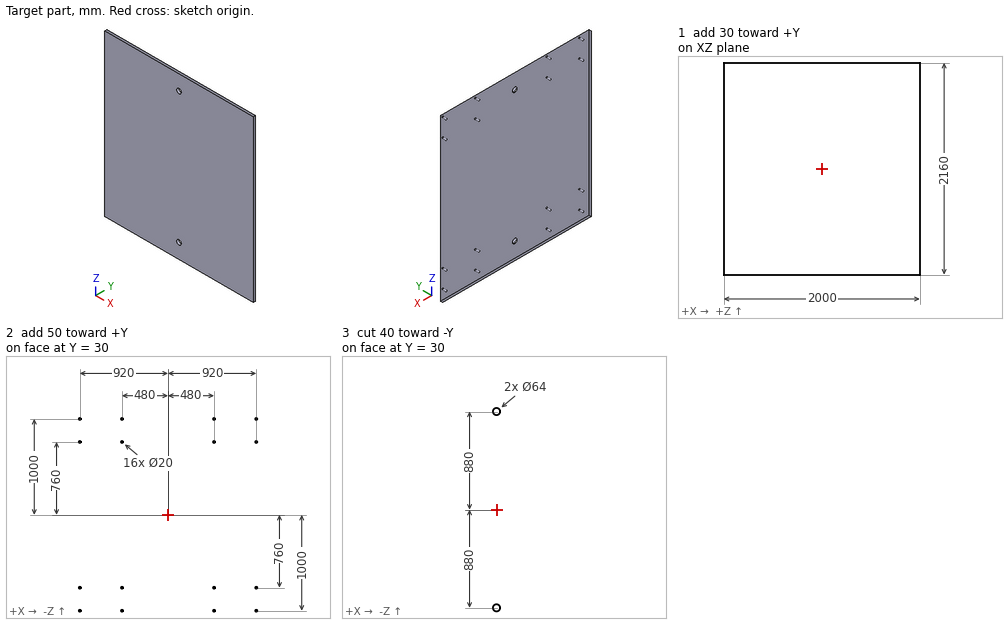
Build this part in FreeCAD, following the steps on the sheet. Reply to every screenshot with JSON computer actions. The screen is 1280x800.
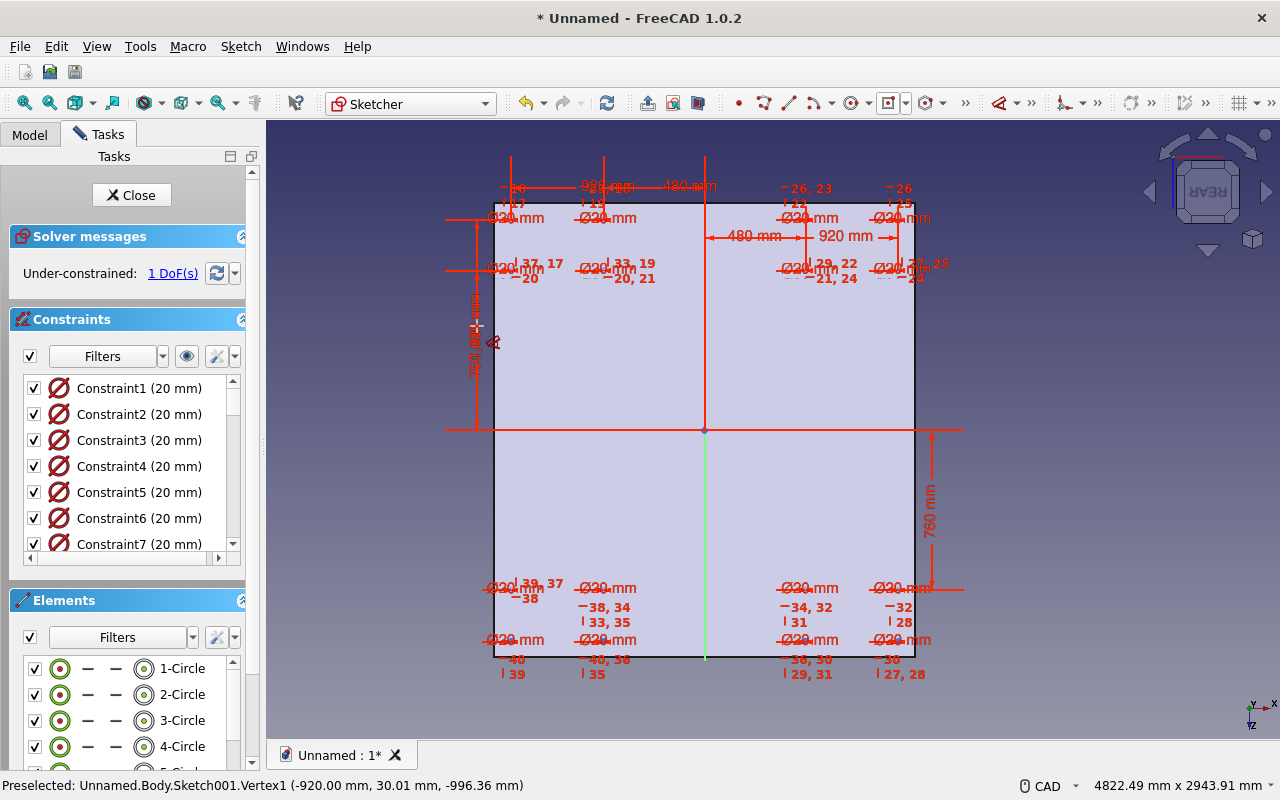
{"action": "left_click", "coordinate": [898, 642]}
{"action": "left_click", "coordinate": [932, 536]}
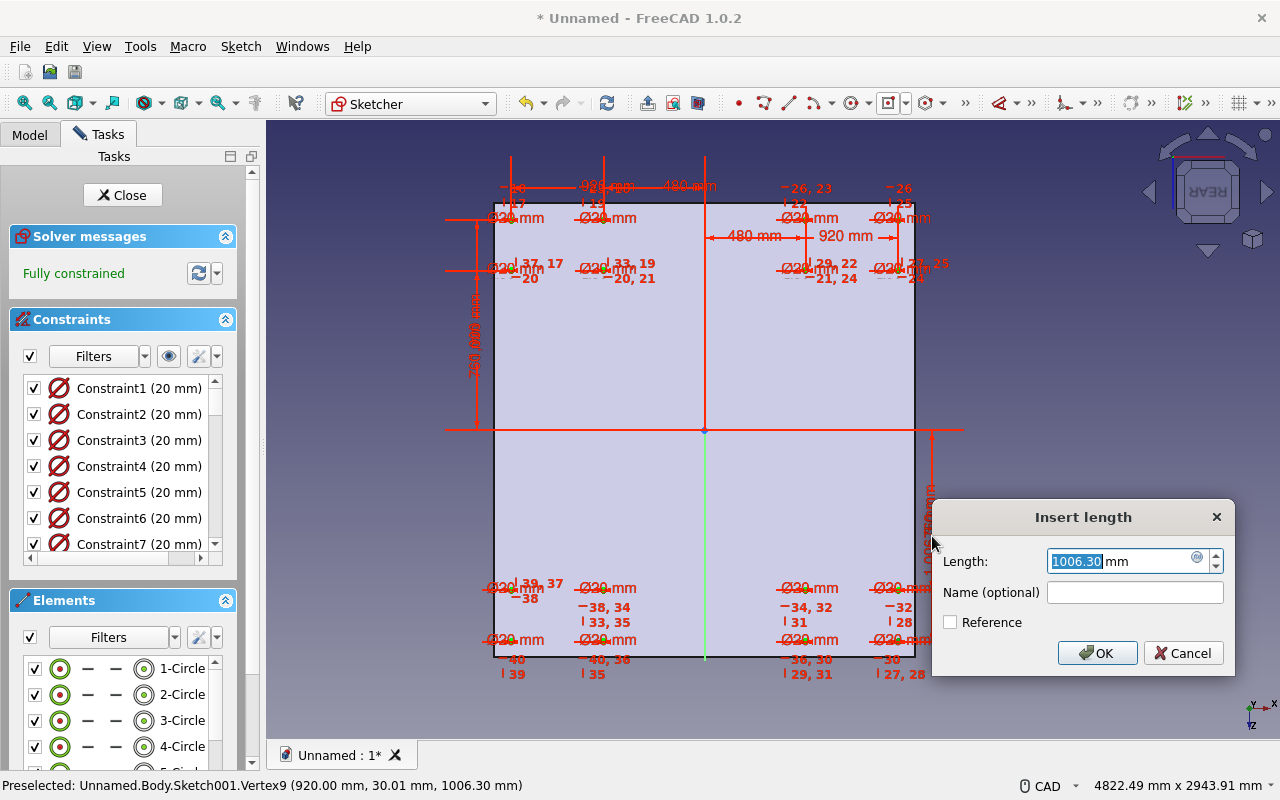
{"action": "type", "text": "1000"}
{"action": "key", "text": "Return"}
{"action": "key", "text": "Escape"}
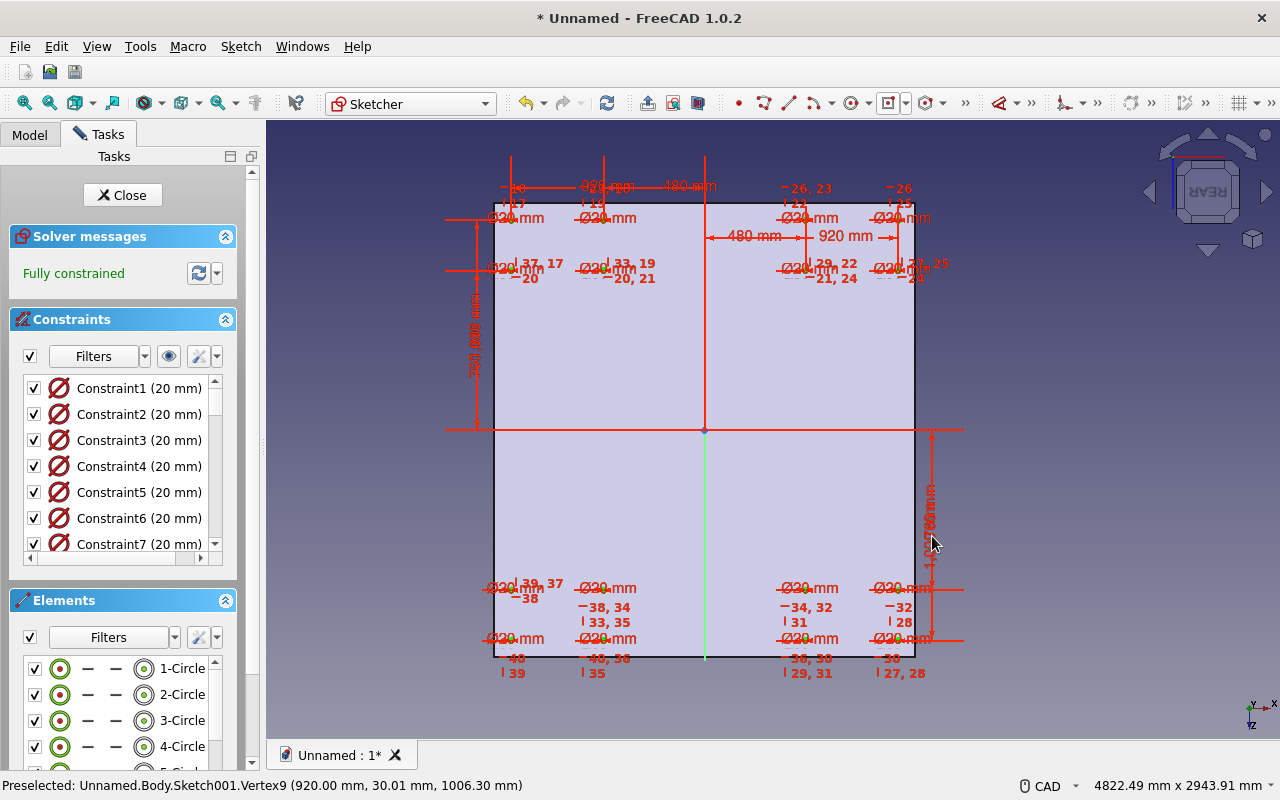
{"action": "left_click", "coordinate": [123, 195]}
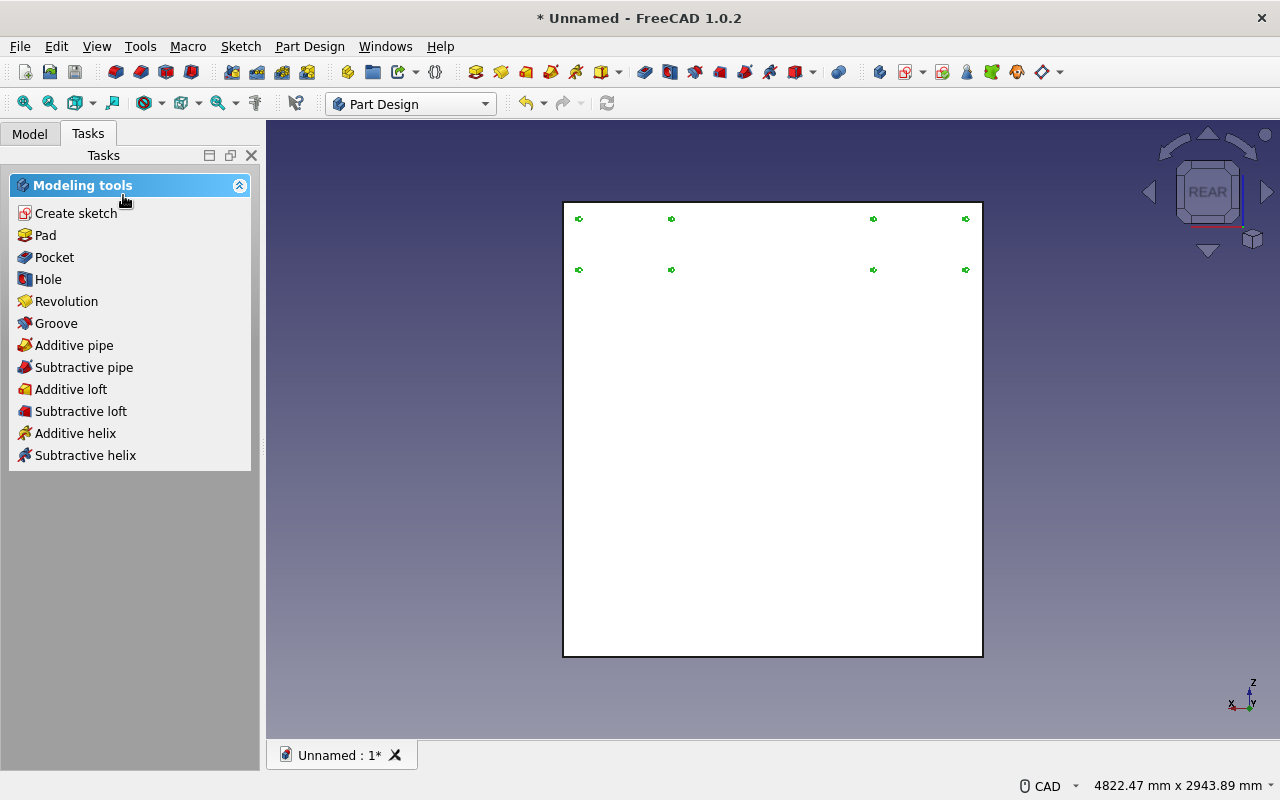
{"action": "left_click", "coordinate": [476, 72]}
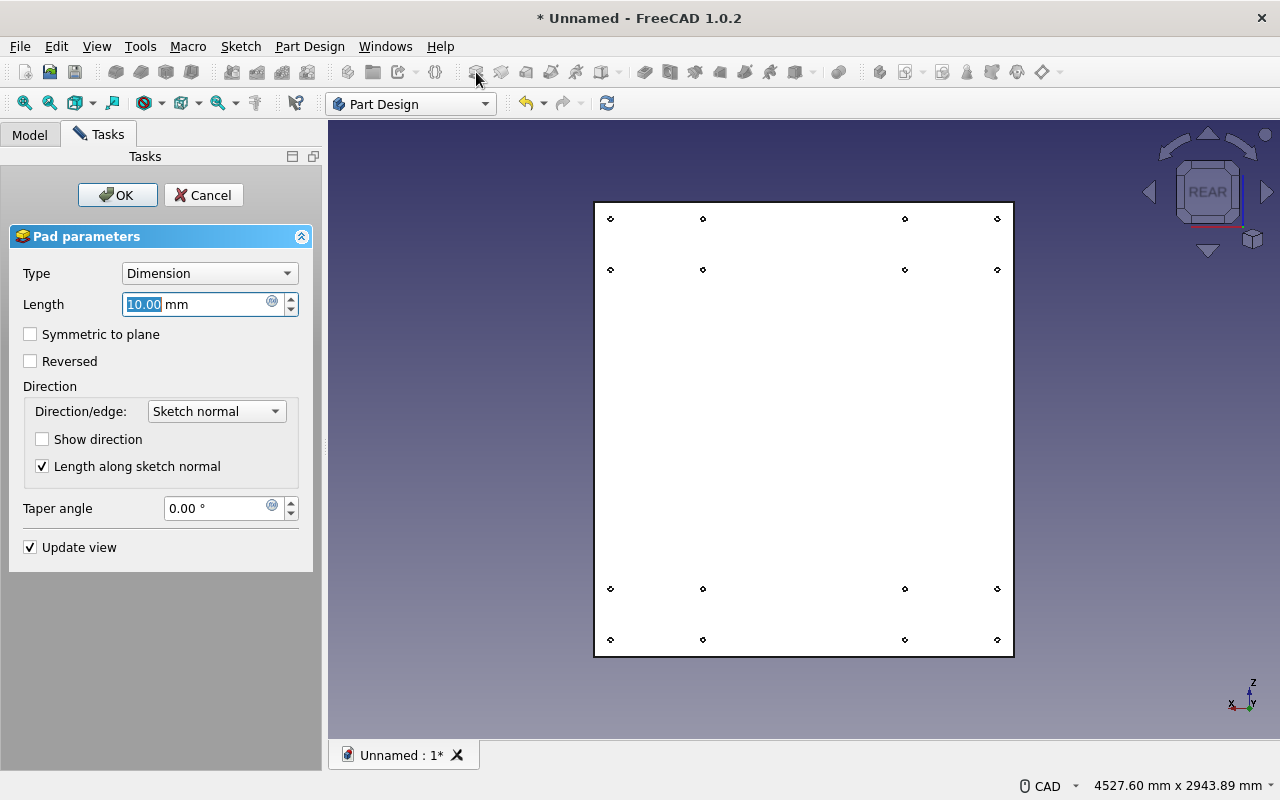
{"action": "type", "text": "50"}
{"action": "key", "text": "Tab"}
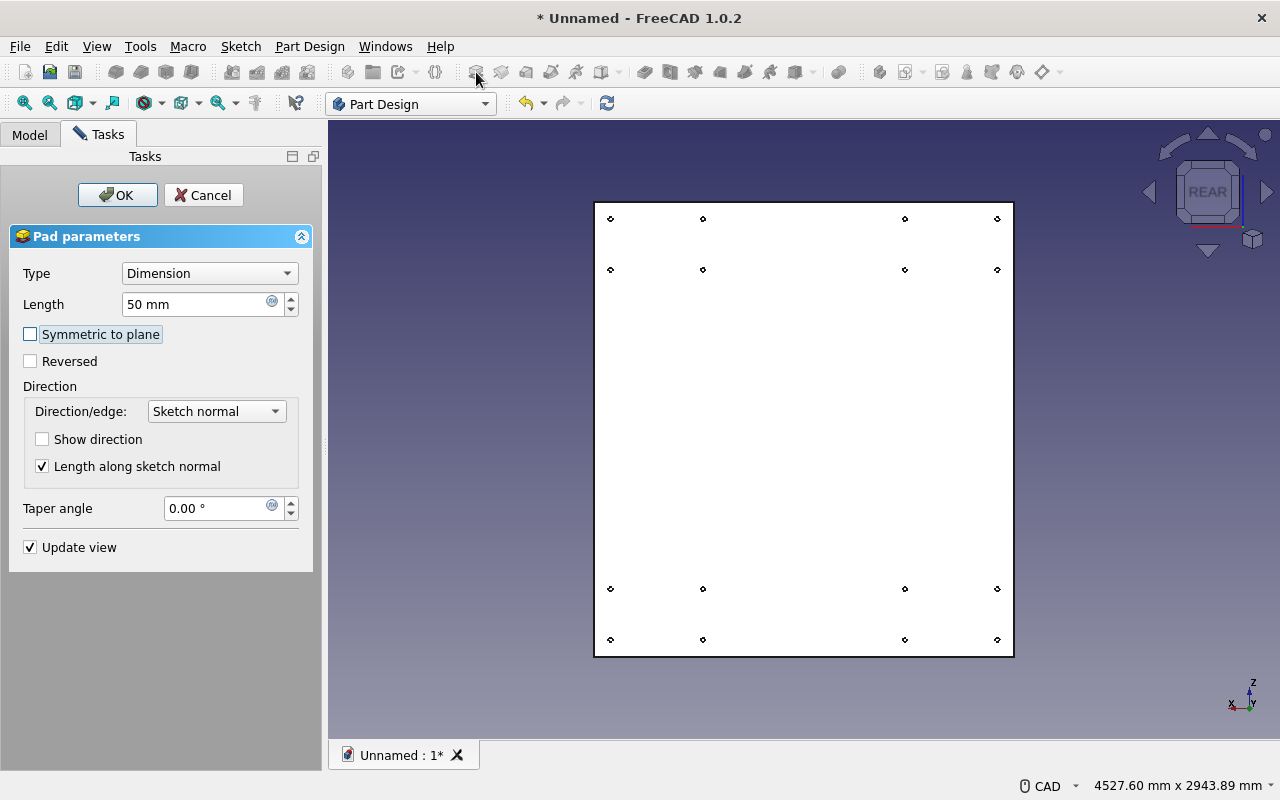
{"action": "left_click", "coordinate": [118, 195]}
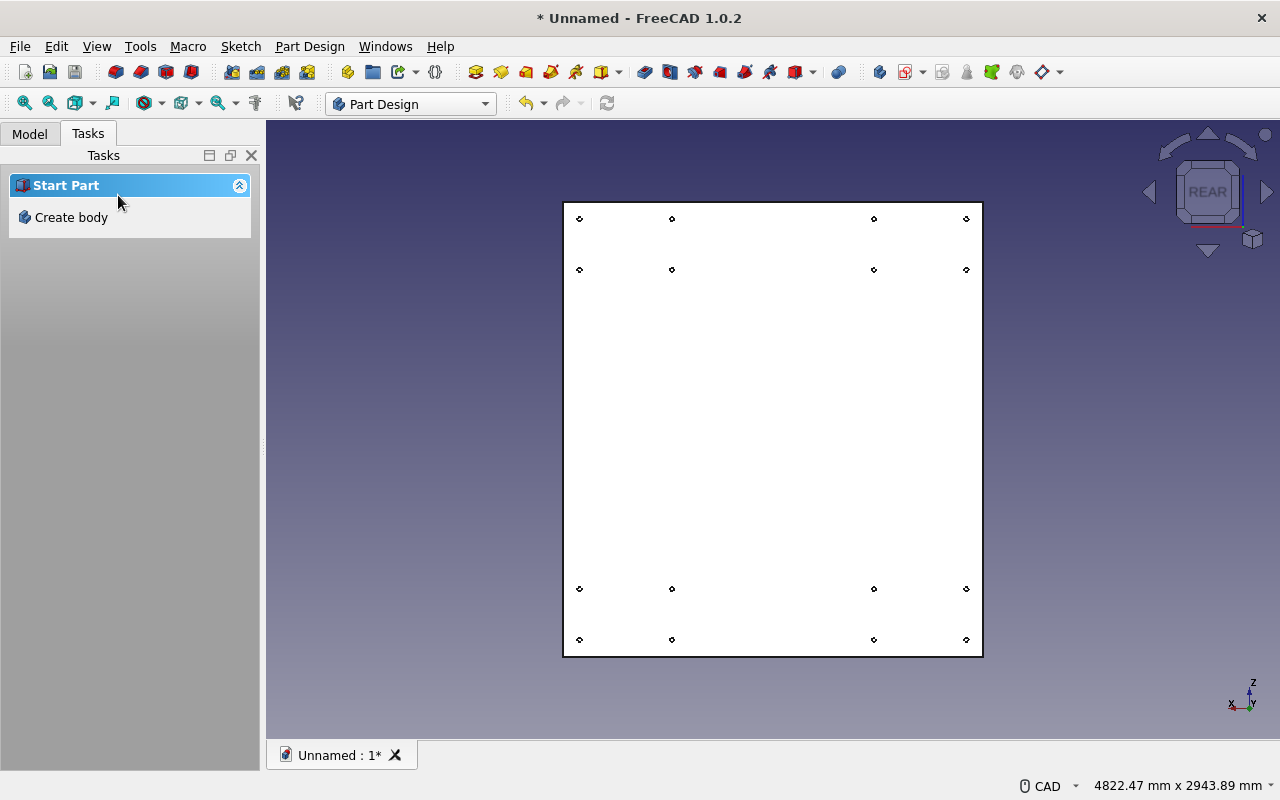
{"action": "left_click", "coordinate": [773, 429]}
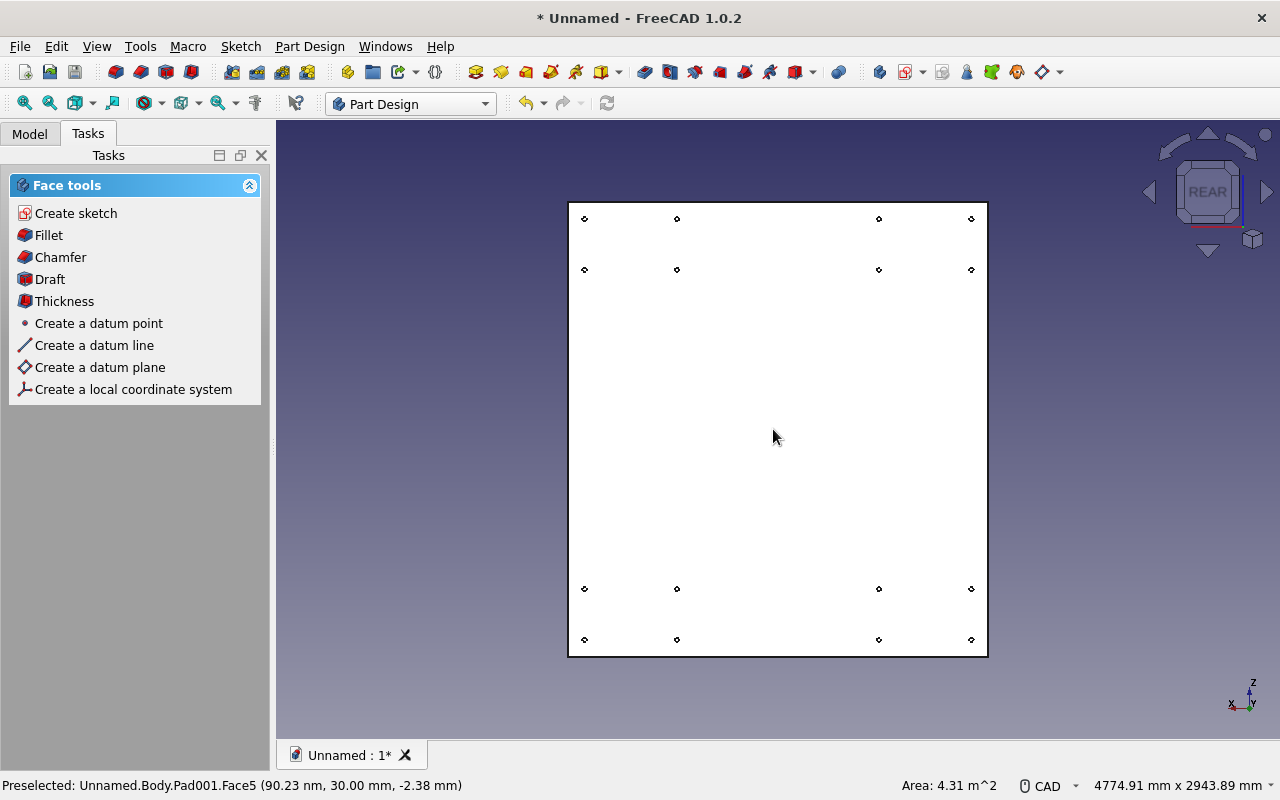
{"action": "left_click", "coordinate": [904, 72]}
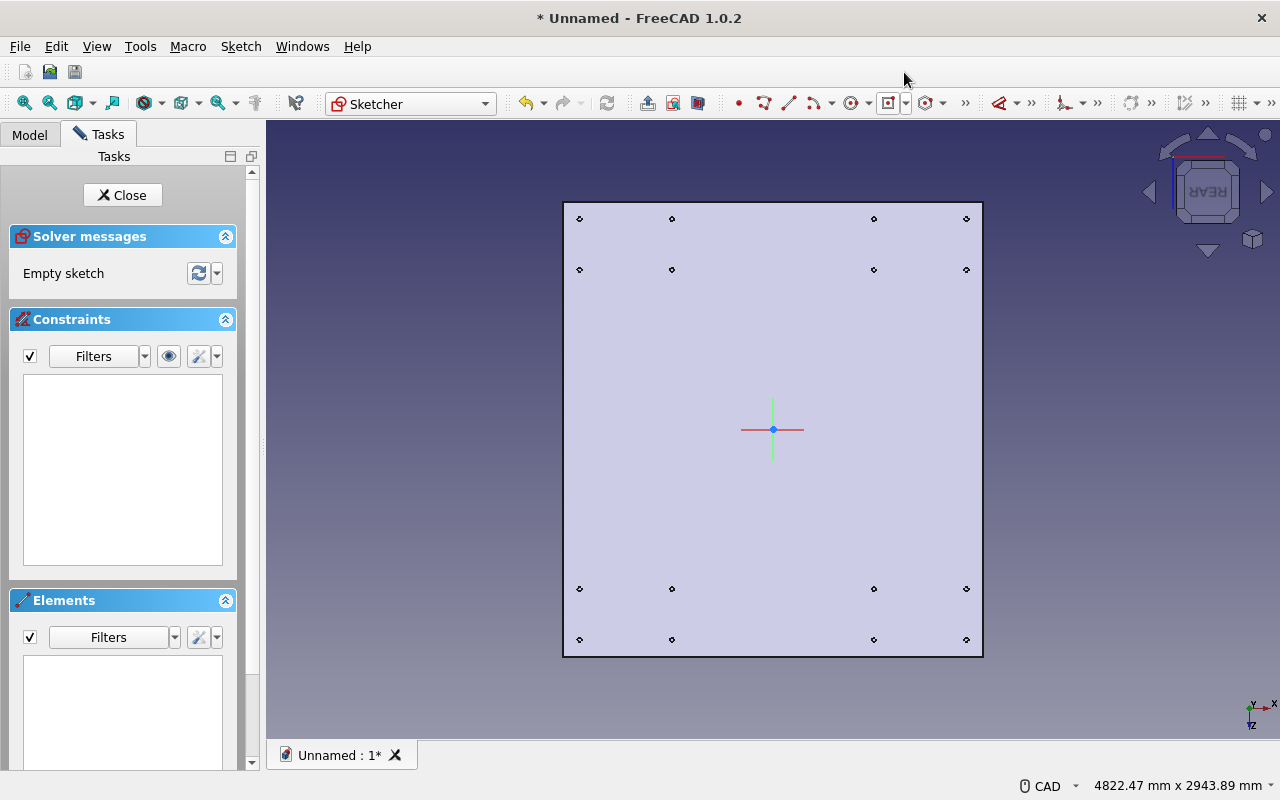
{"action": "left_click", "coordinate": [698, 104]}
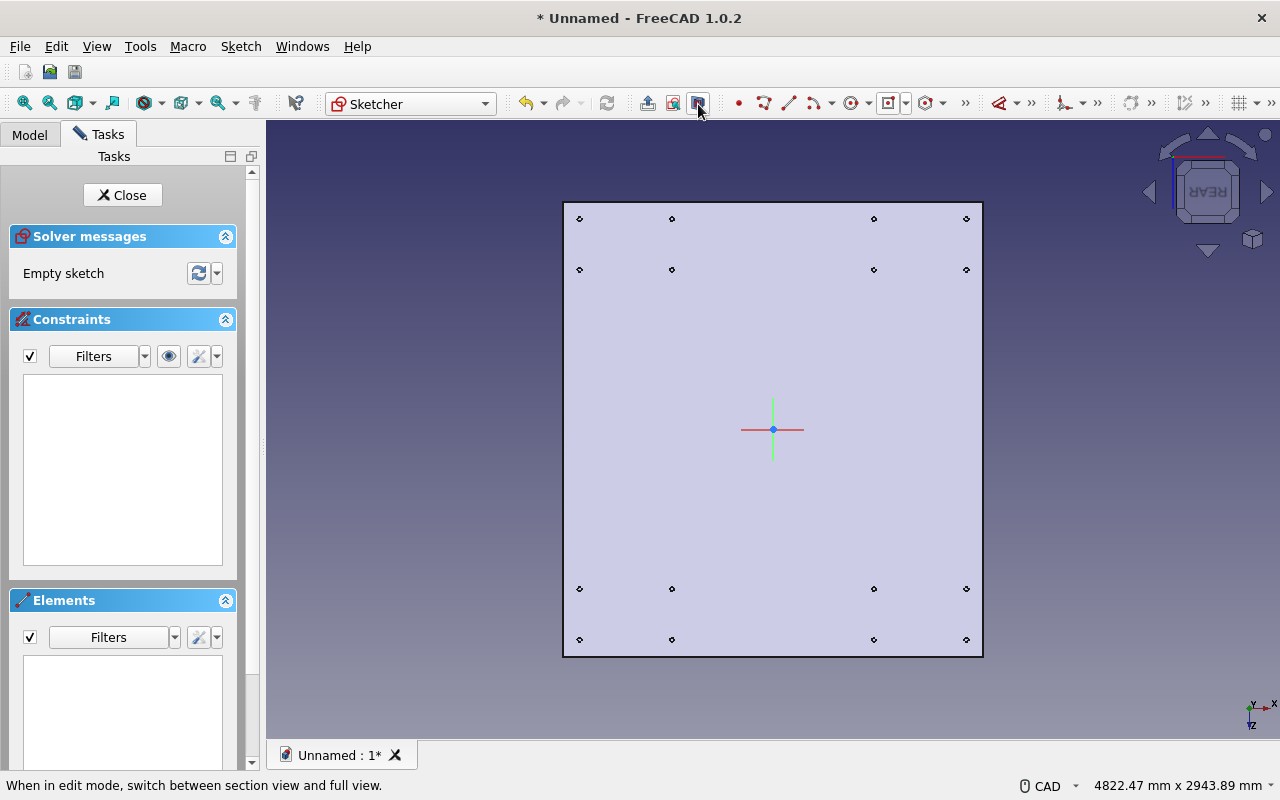
{"action": "left_click", "coordinate": [850, 104]}